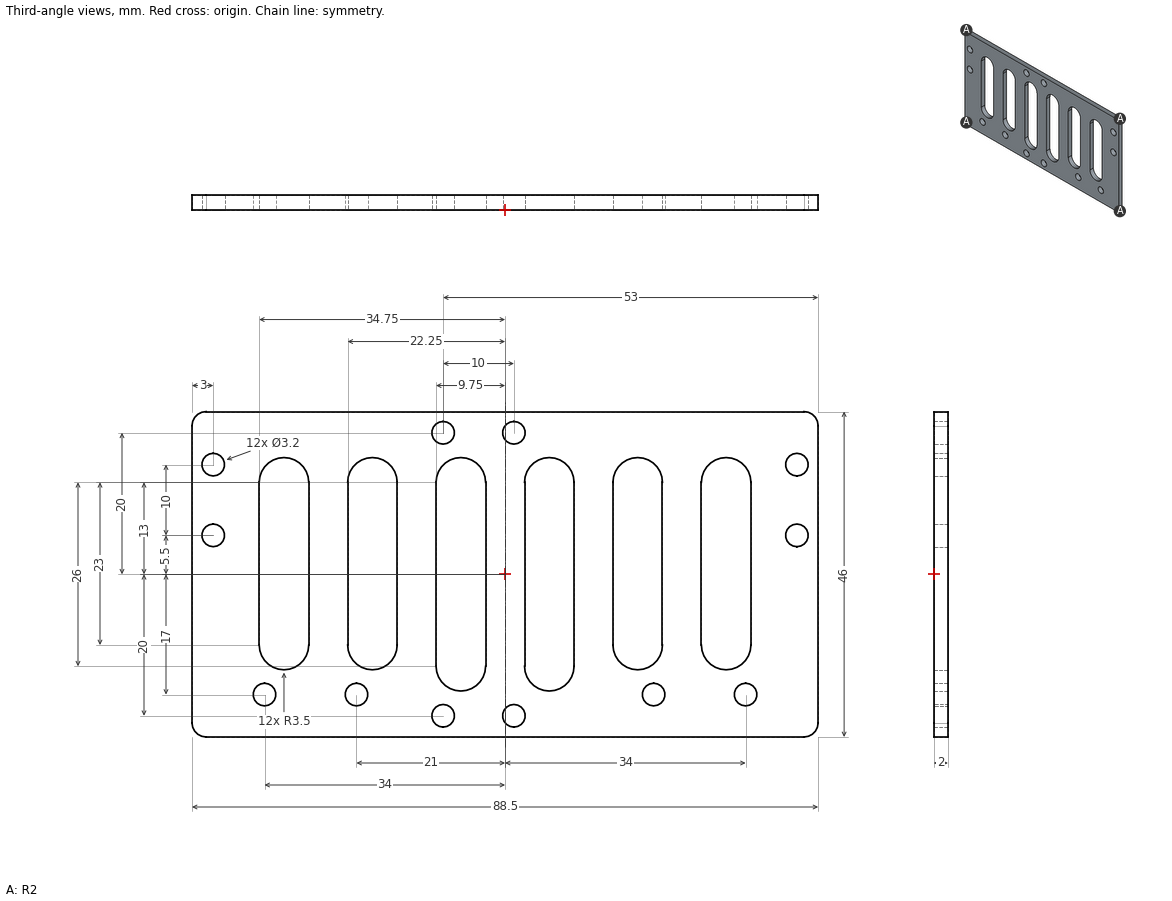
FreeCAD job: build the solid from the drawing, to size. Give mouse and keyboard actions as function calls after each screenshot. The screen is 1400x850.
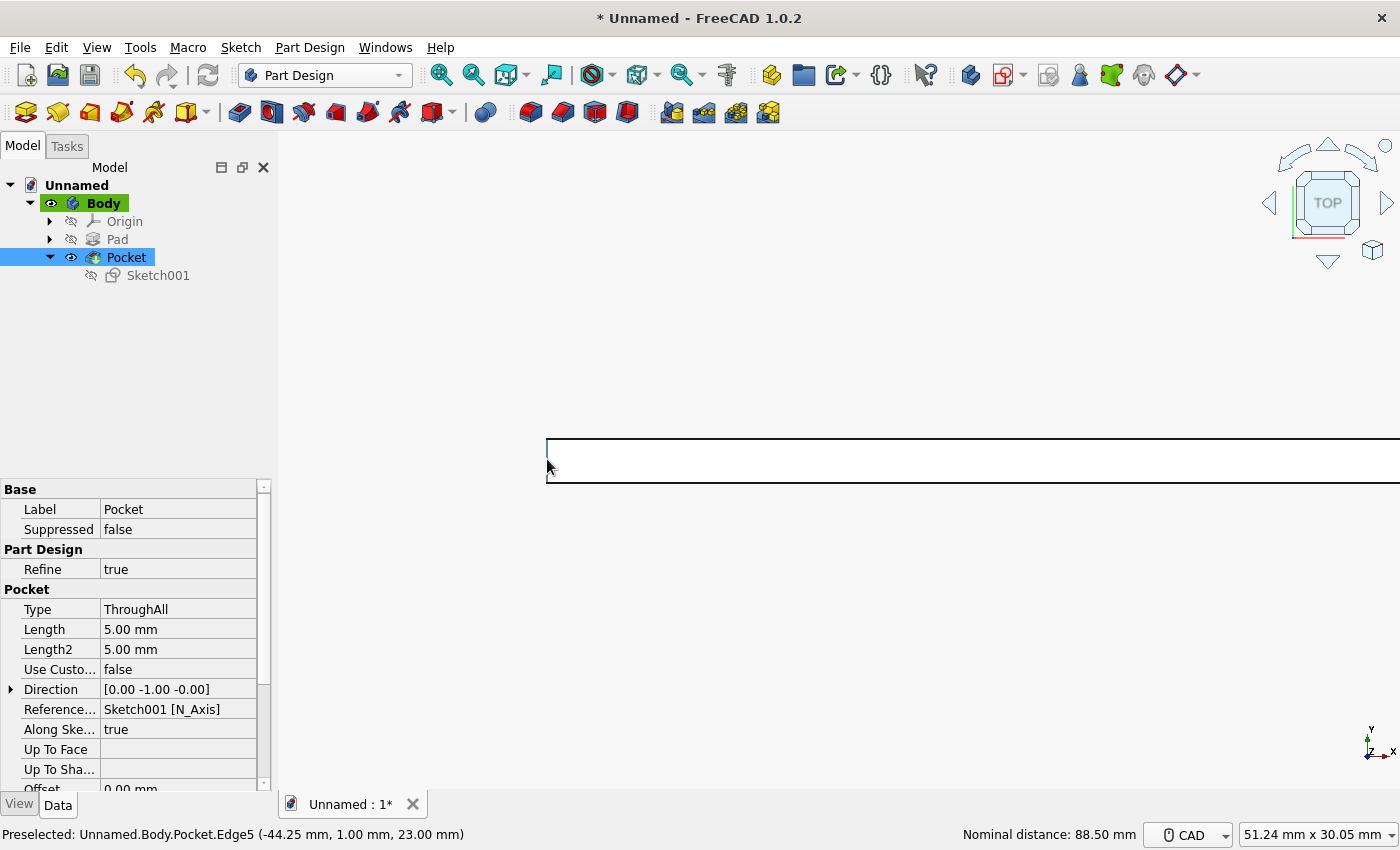
click(442, 76)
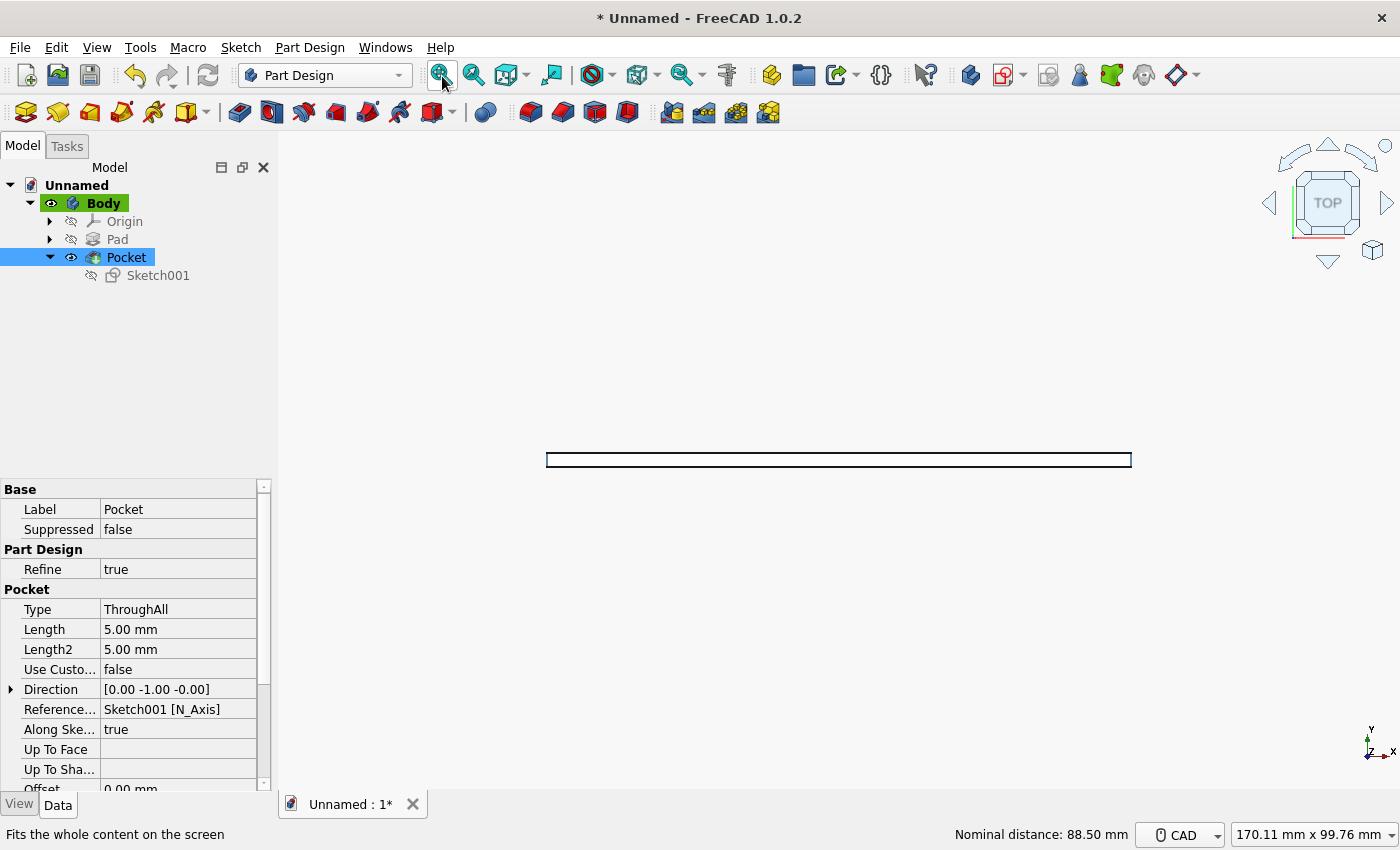
key(1)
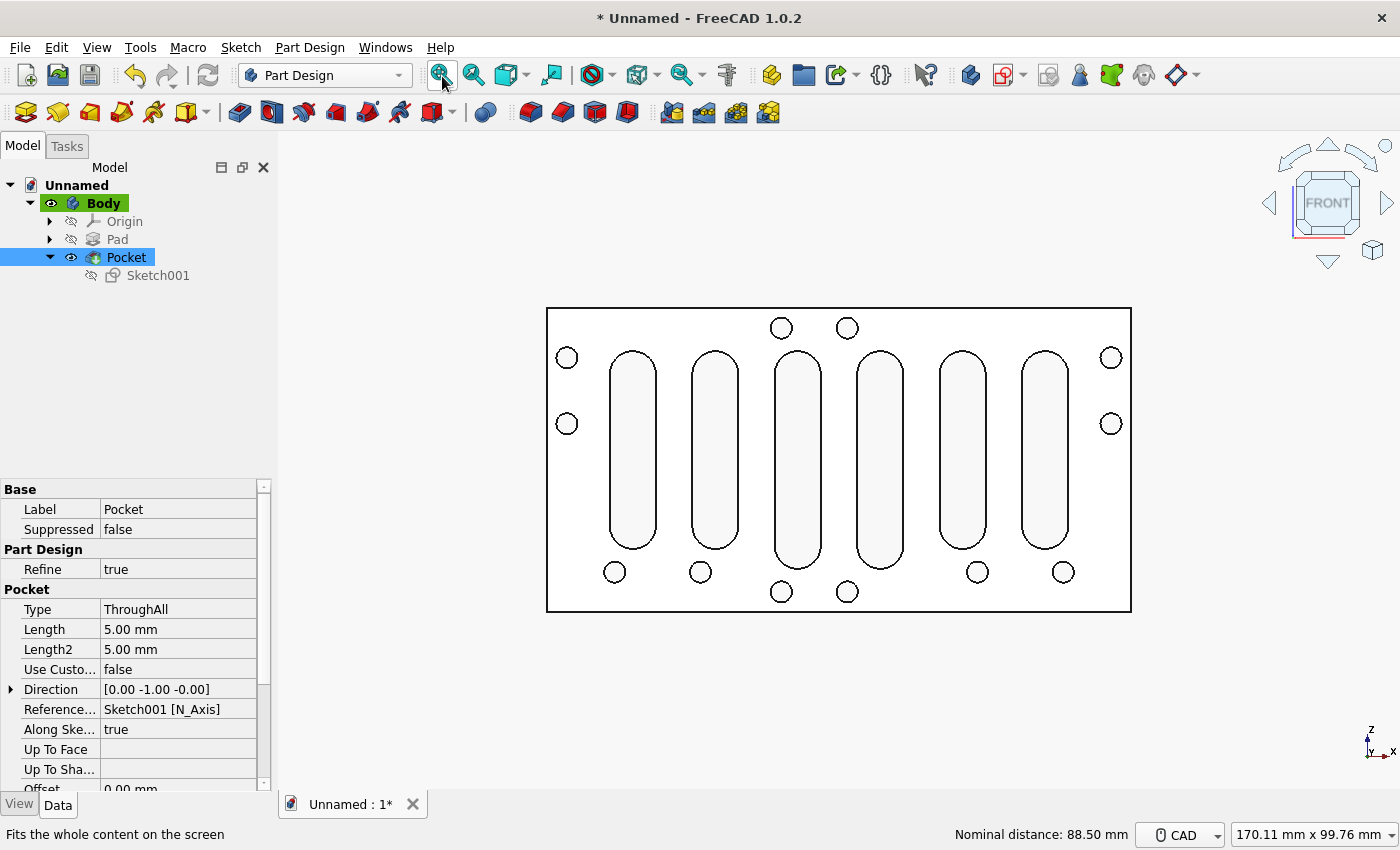
scroll(547, 611, up, 6)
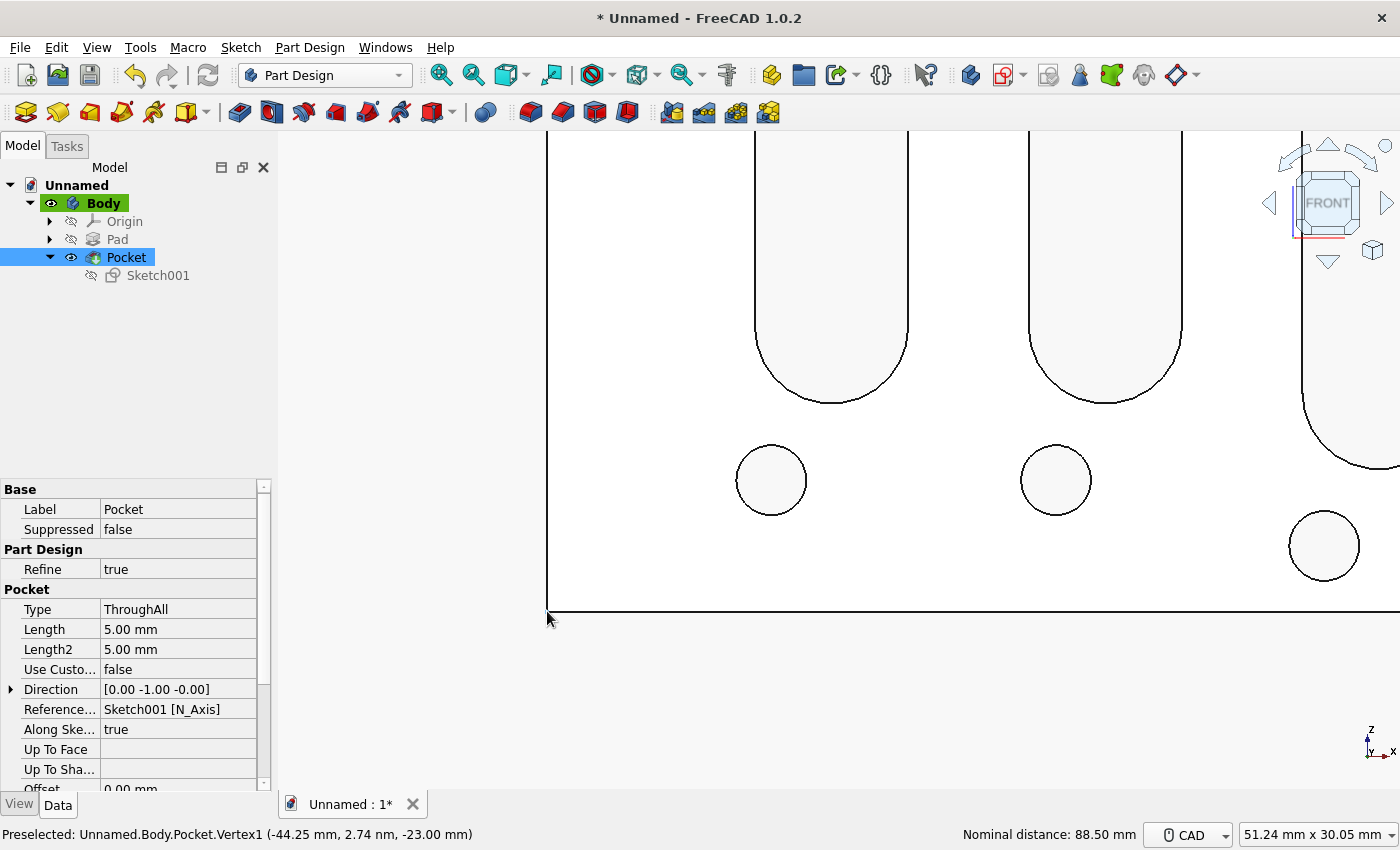
click(442, 76)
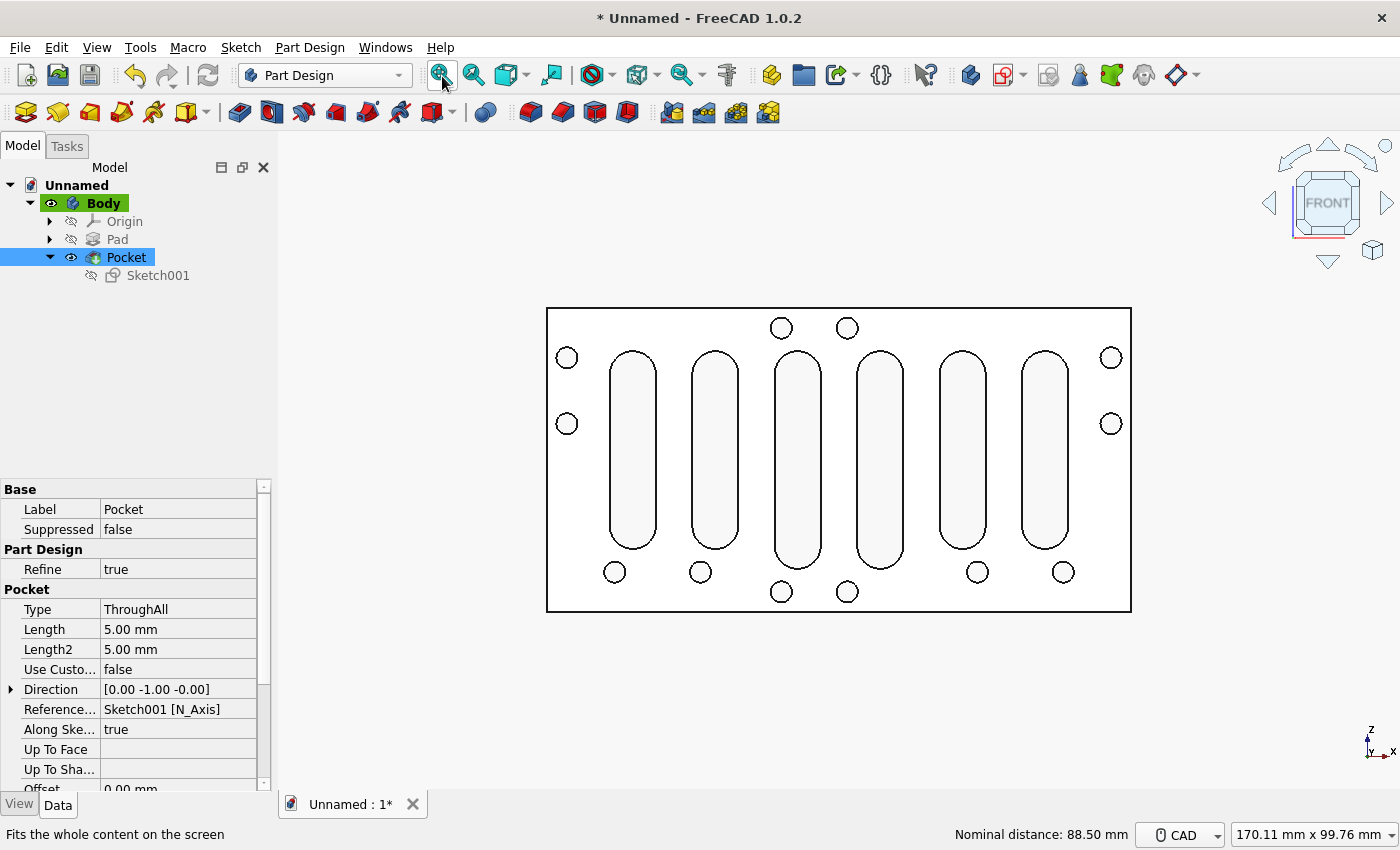
key(3)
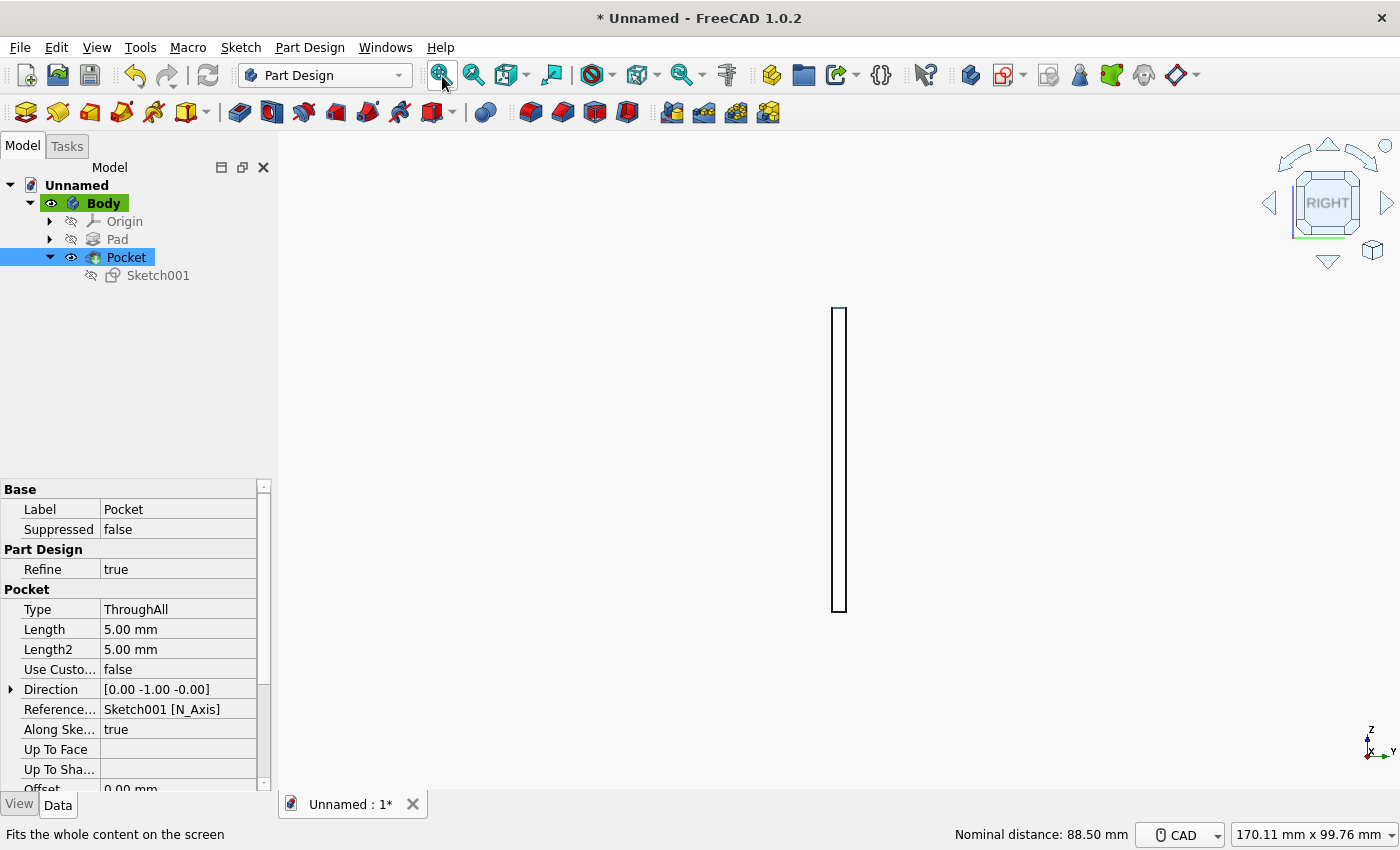
click(839, 611, ctrl)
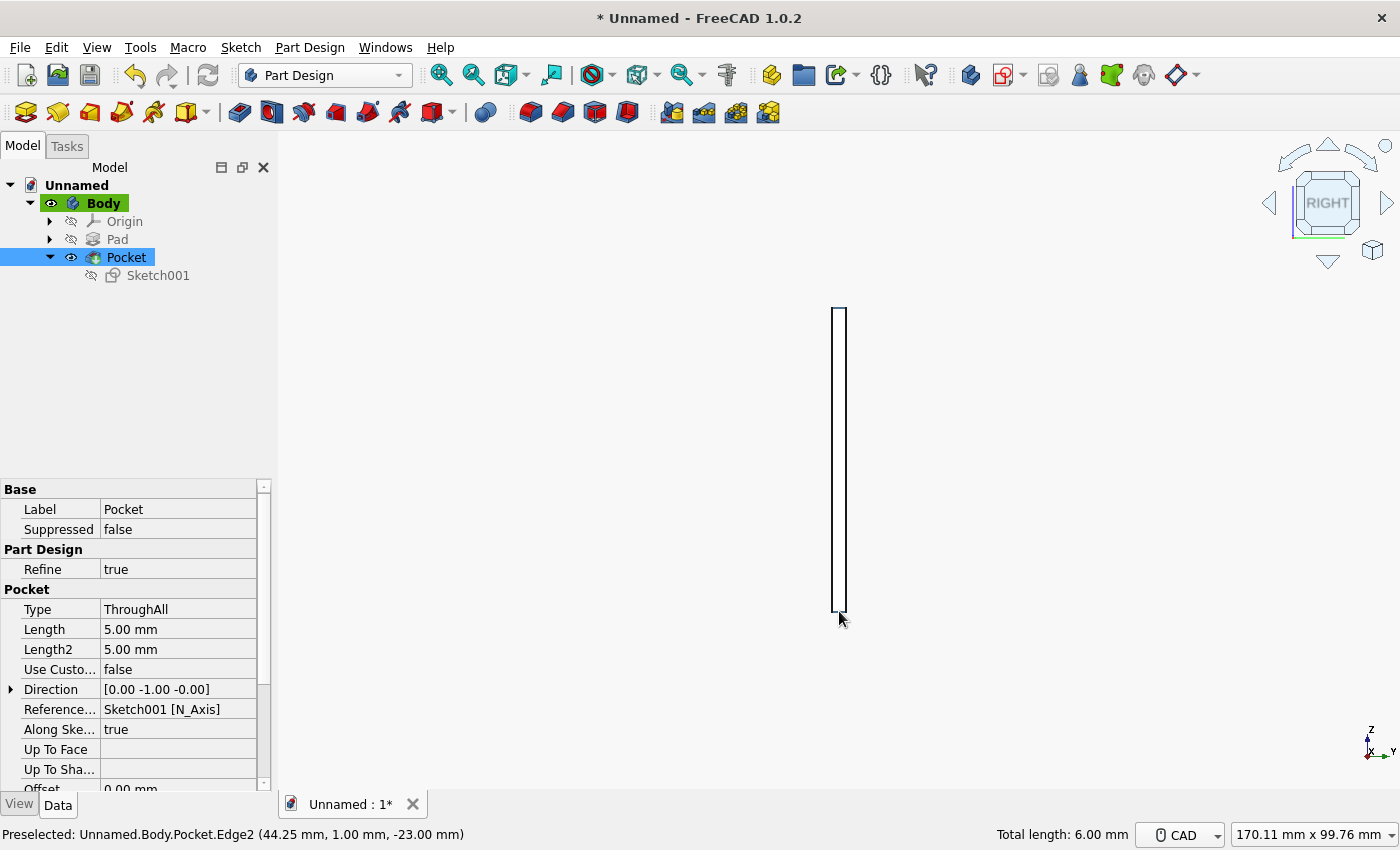
scroll(839, 611, up, 6)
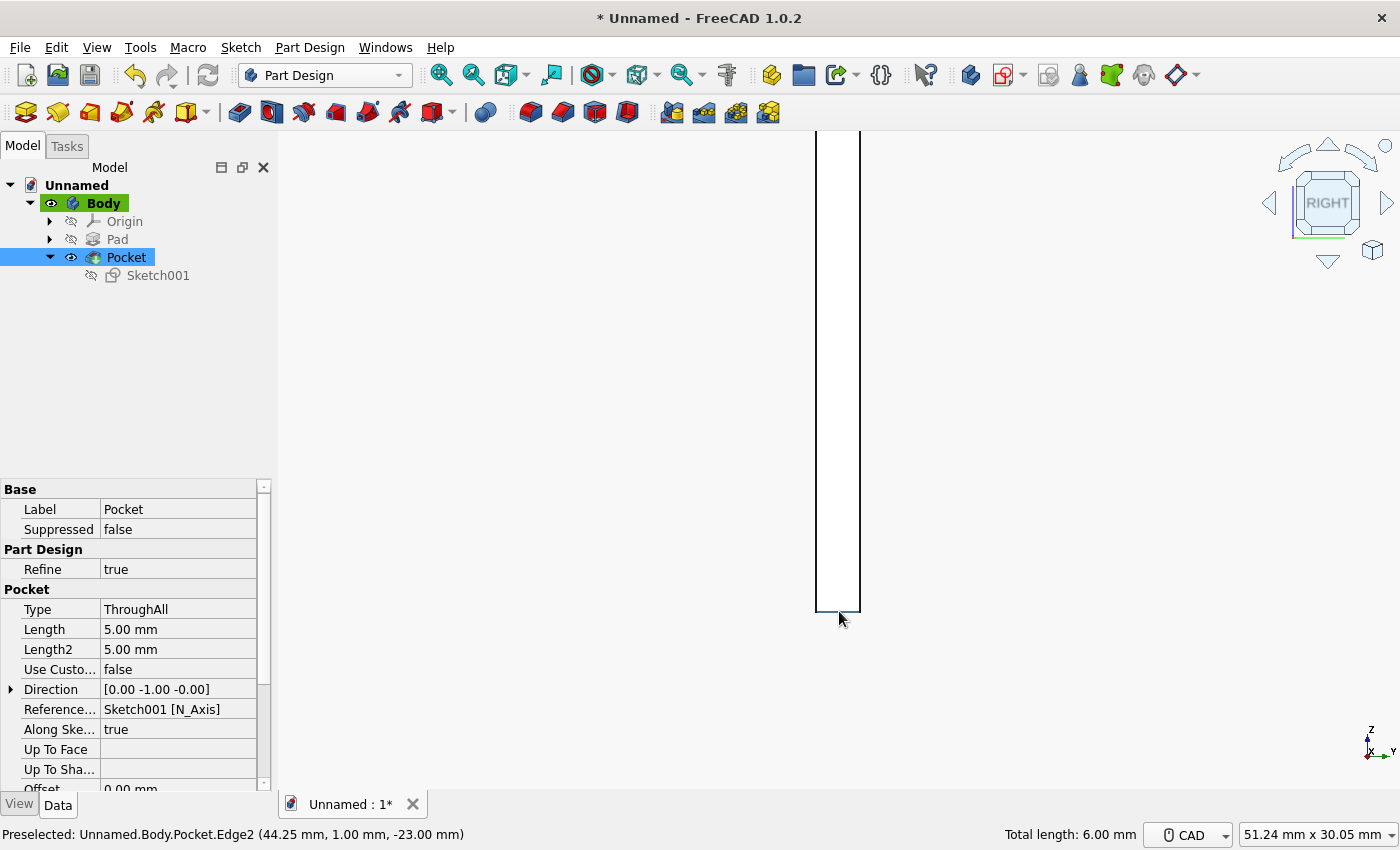
click(442, 76)